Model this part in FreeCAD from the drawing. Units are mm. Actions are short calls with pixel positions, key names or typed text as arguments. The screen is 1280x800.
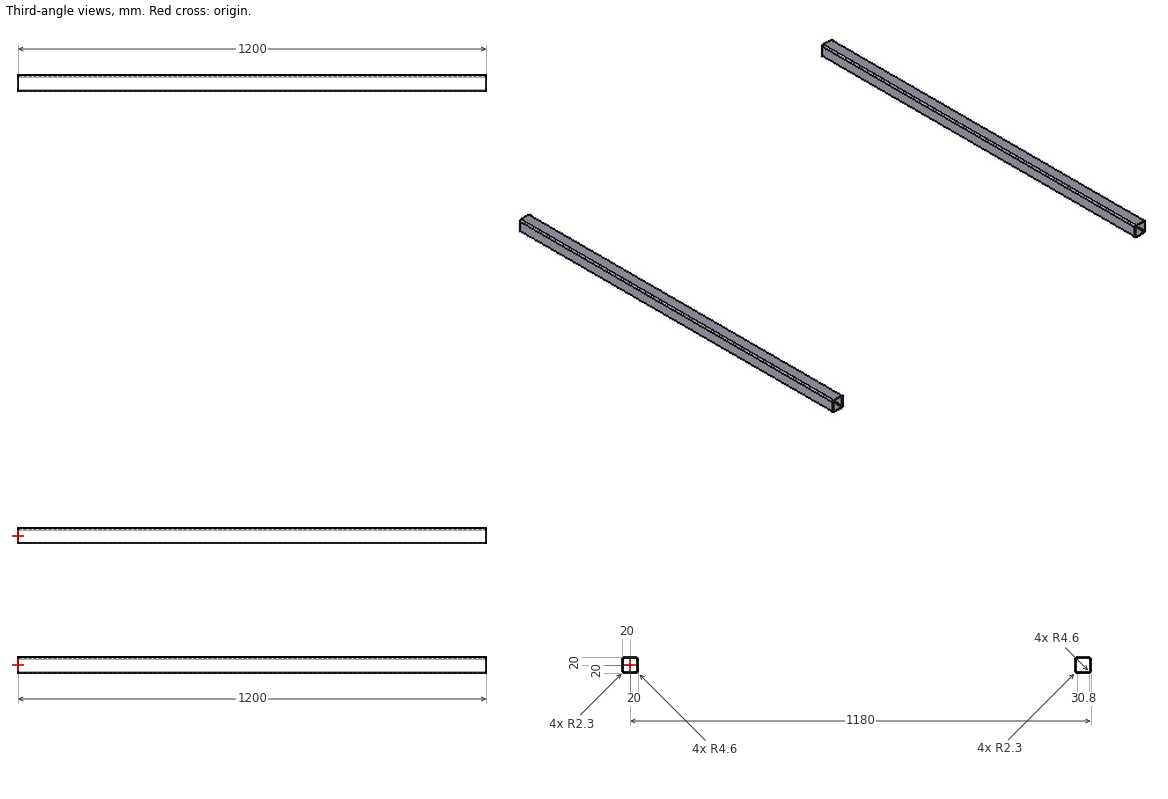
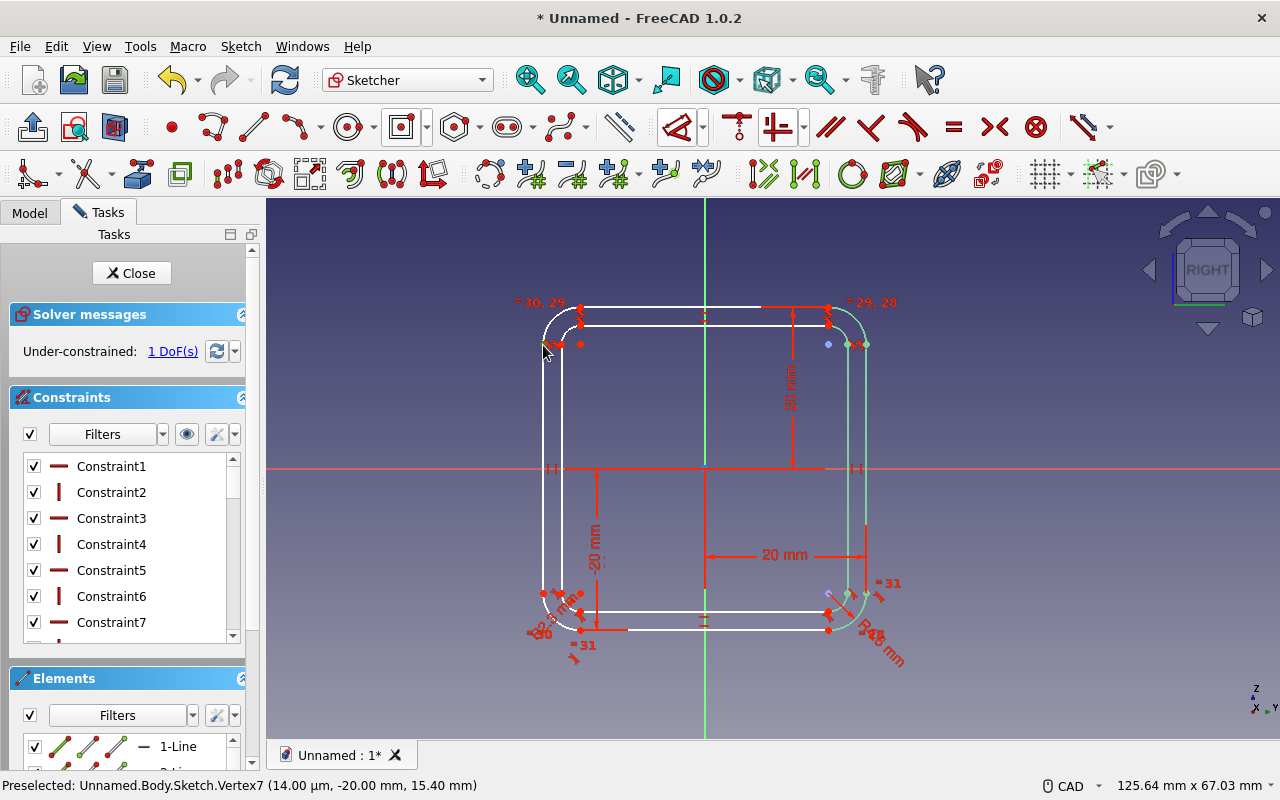
key(l)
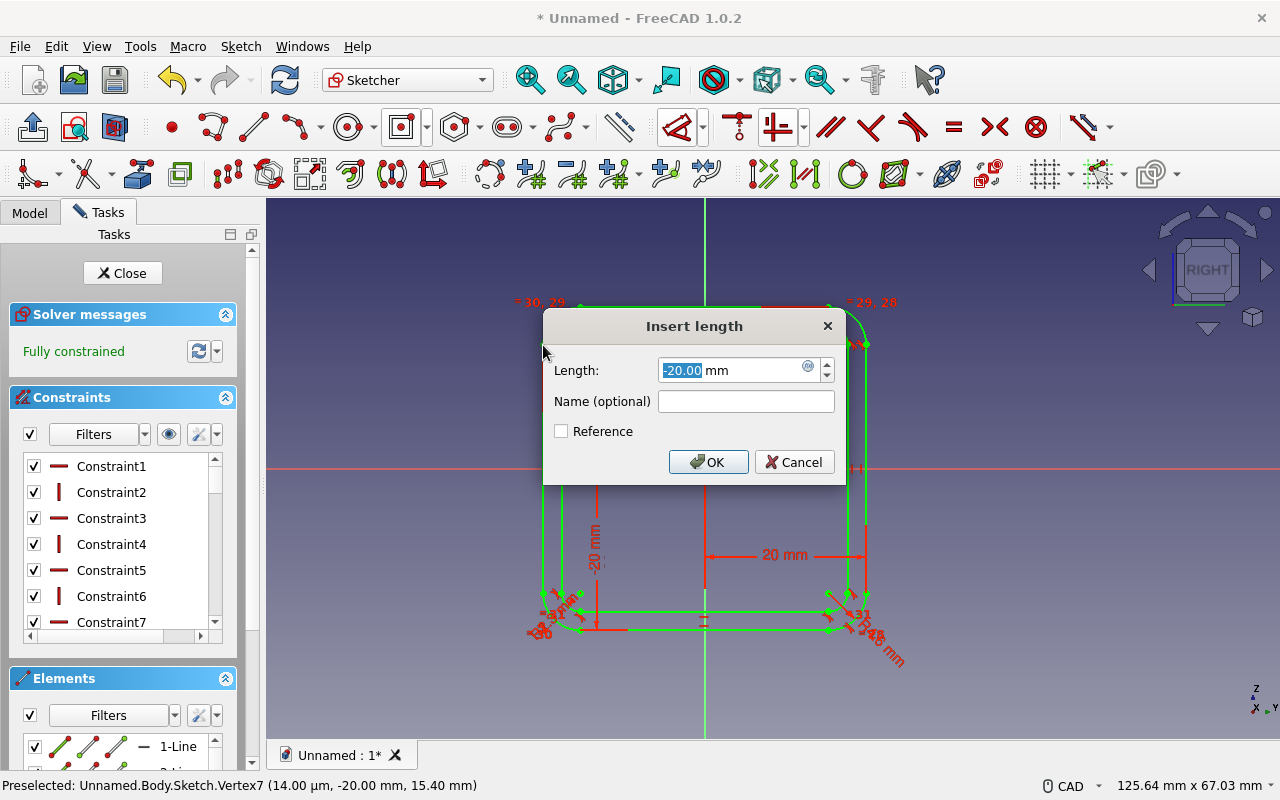
text(-20)
key(Return)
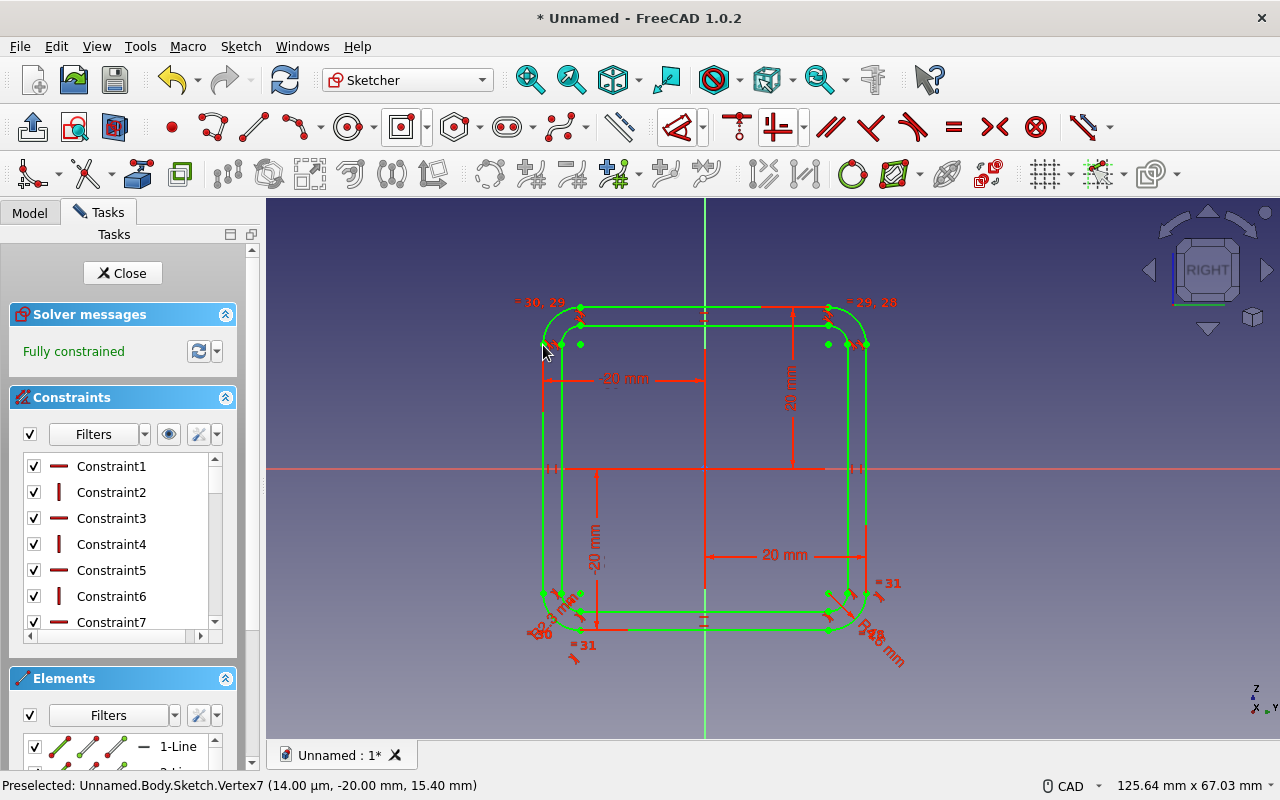
click(123, 273)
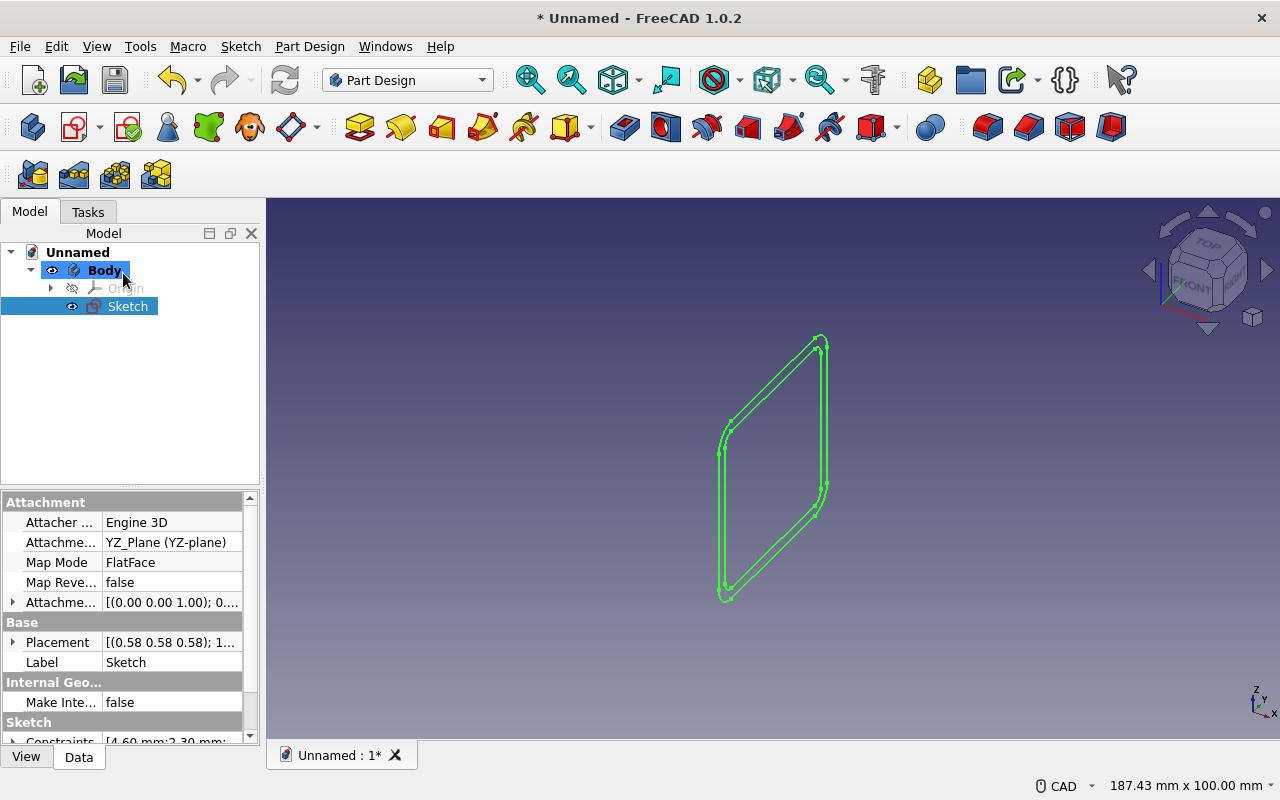
click(360, 128)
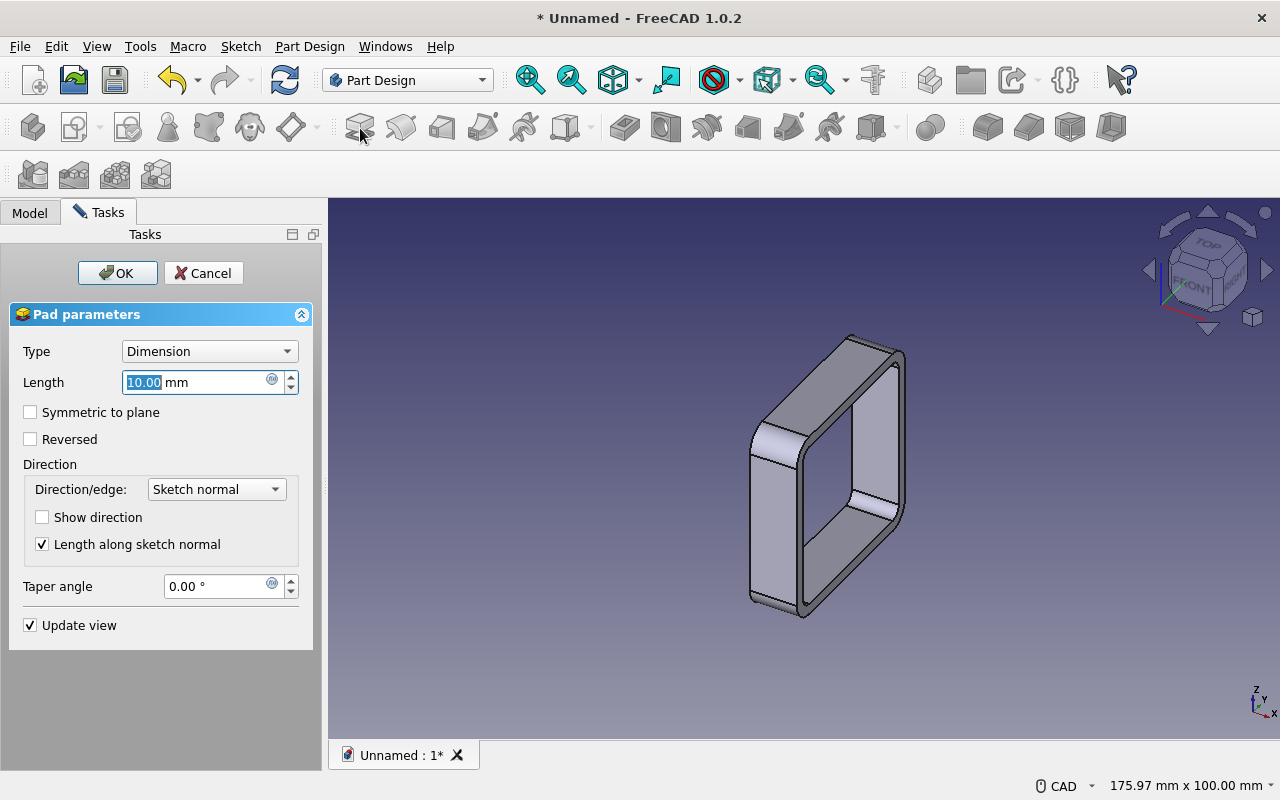
text(1200)
key(Tab)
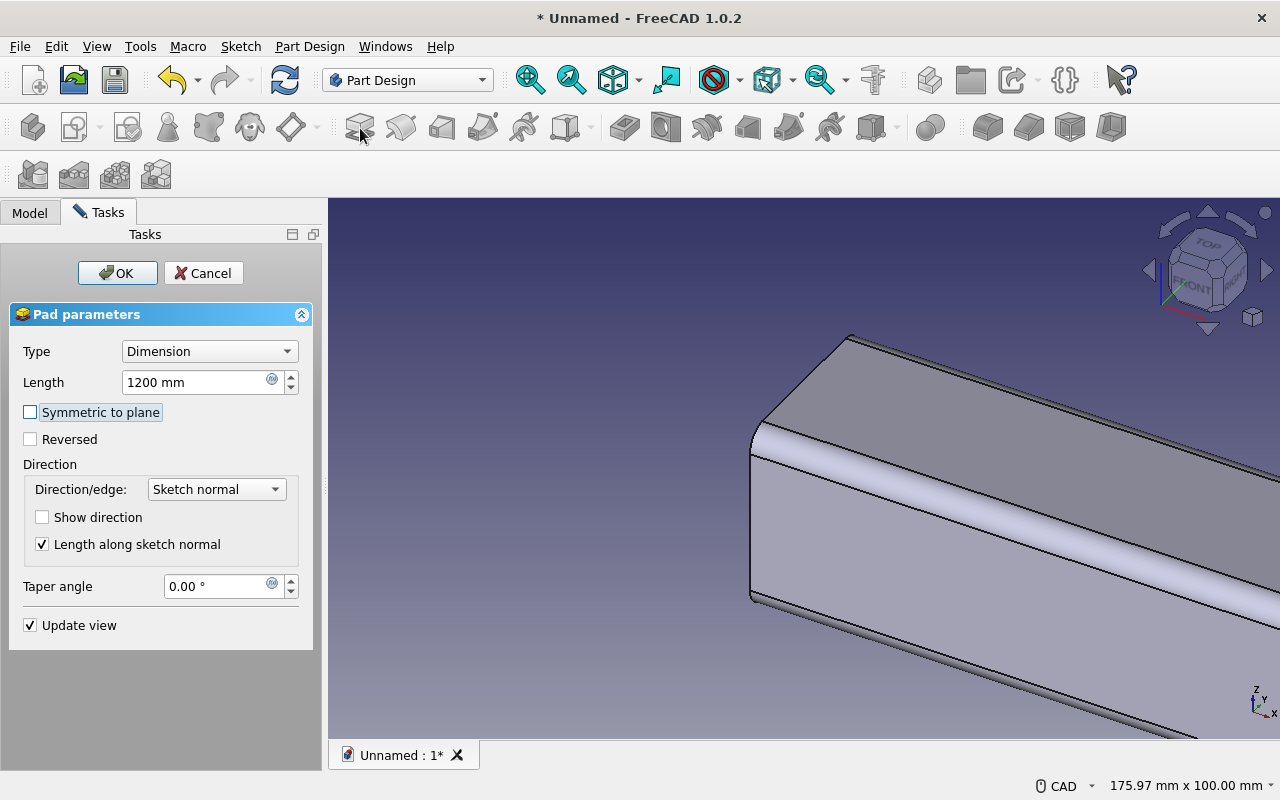
click(118, 273)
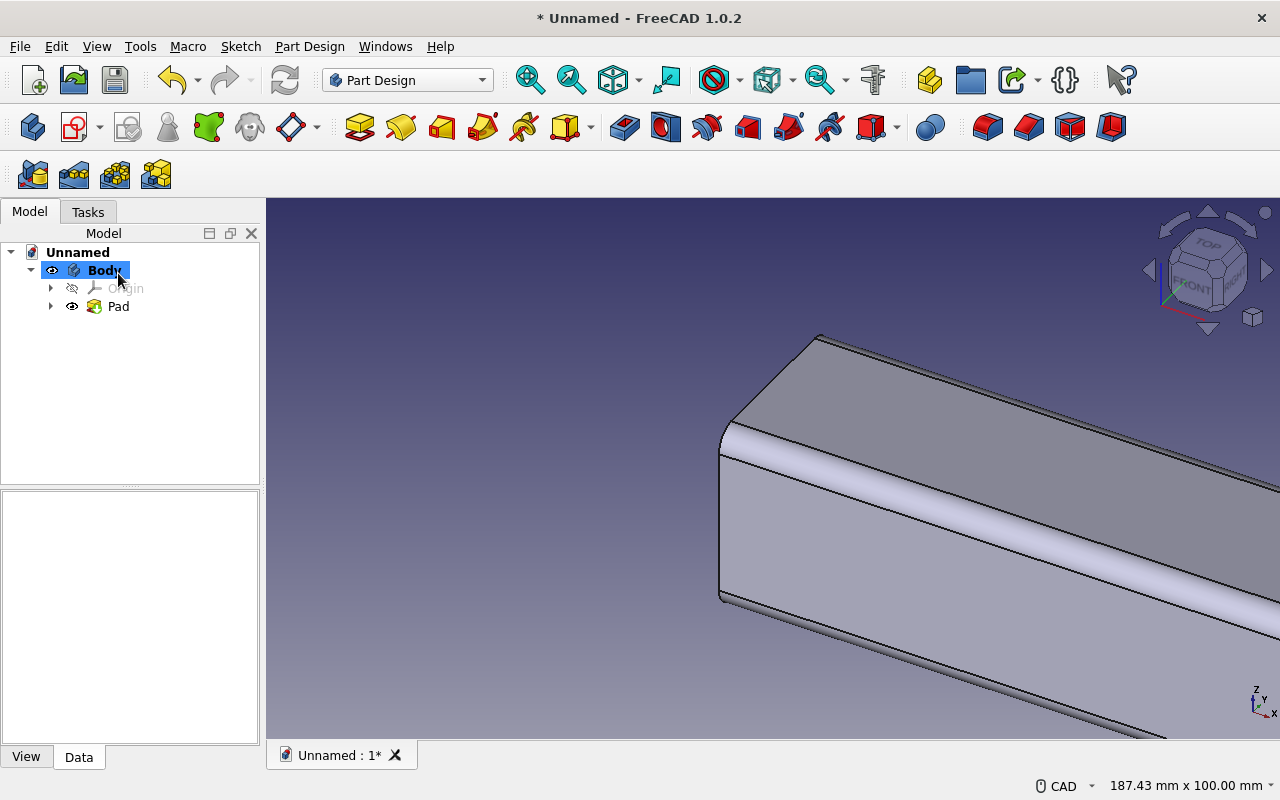
key(v)
key(f)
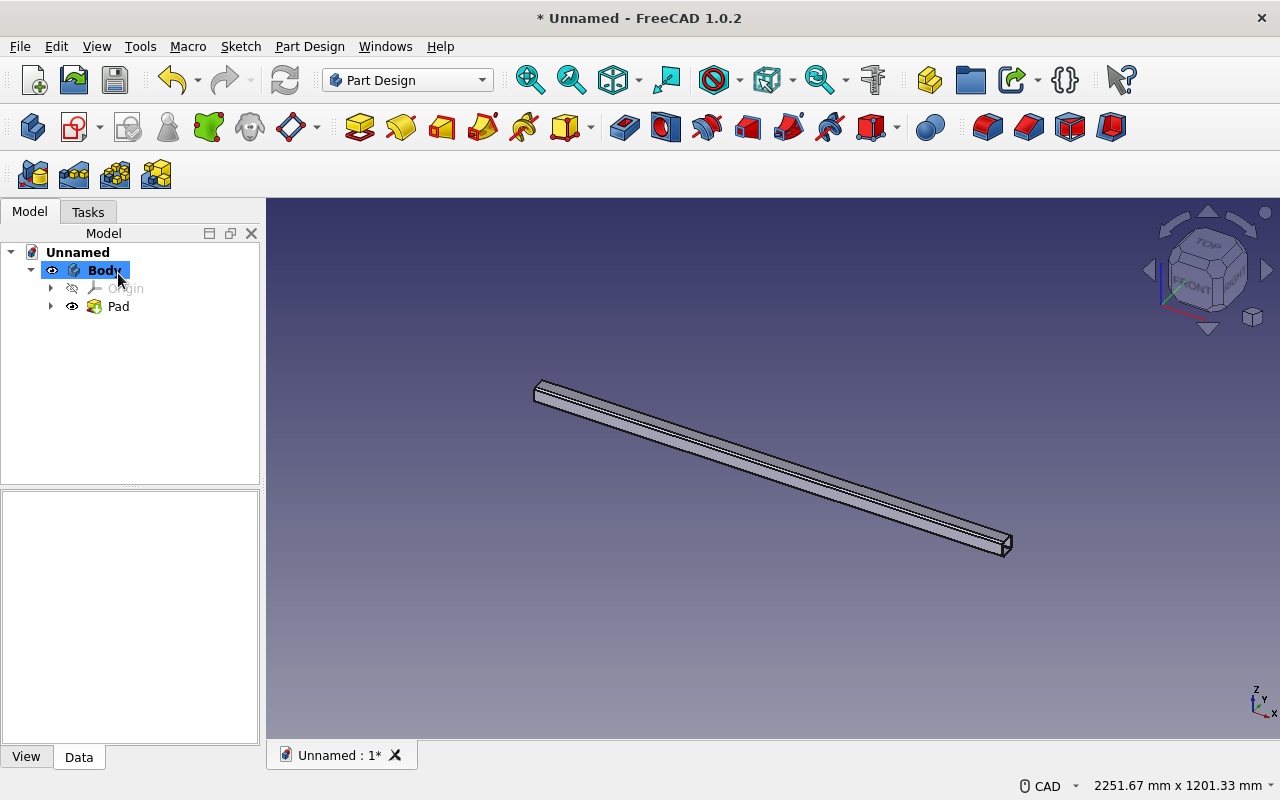
click(33, 128)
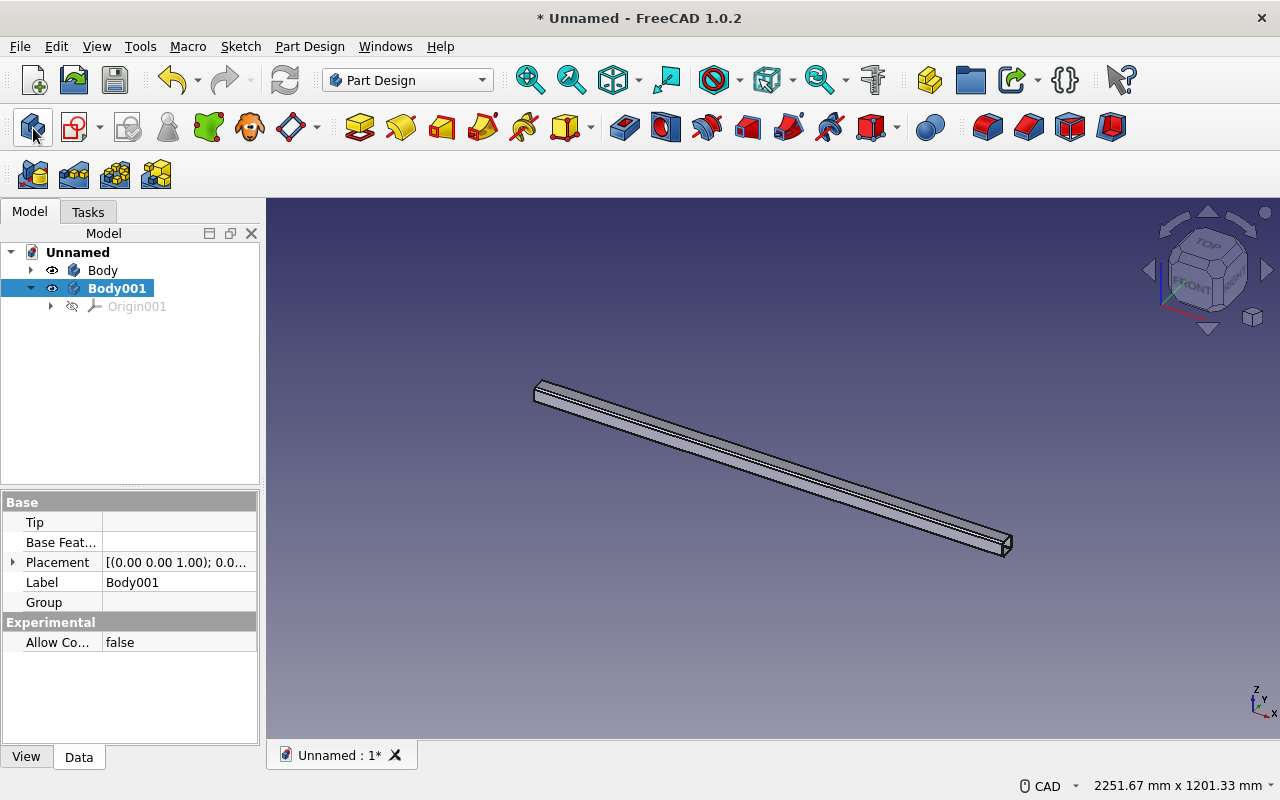
click(306, 699)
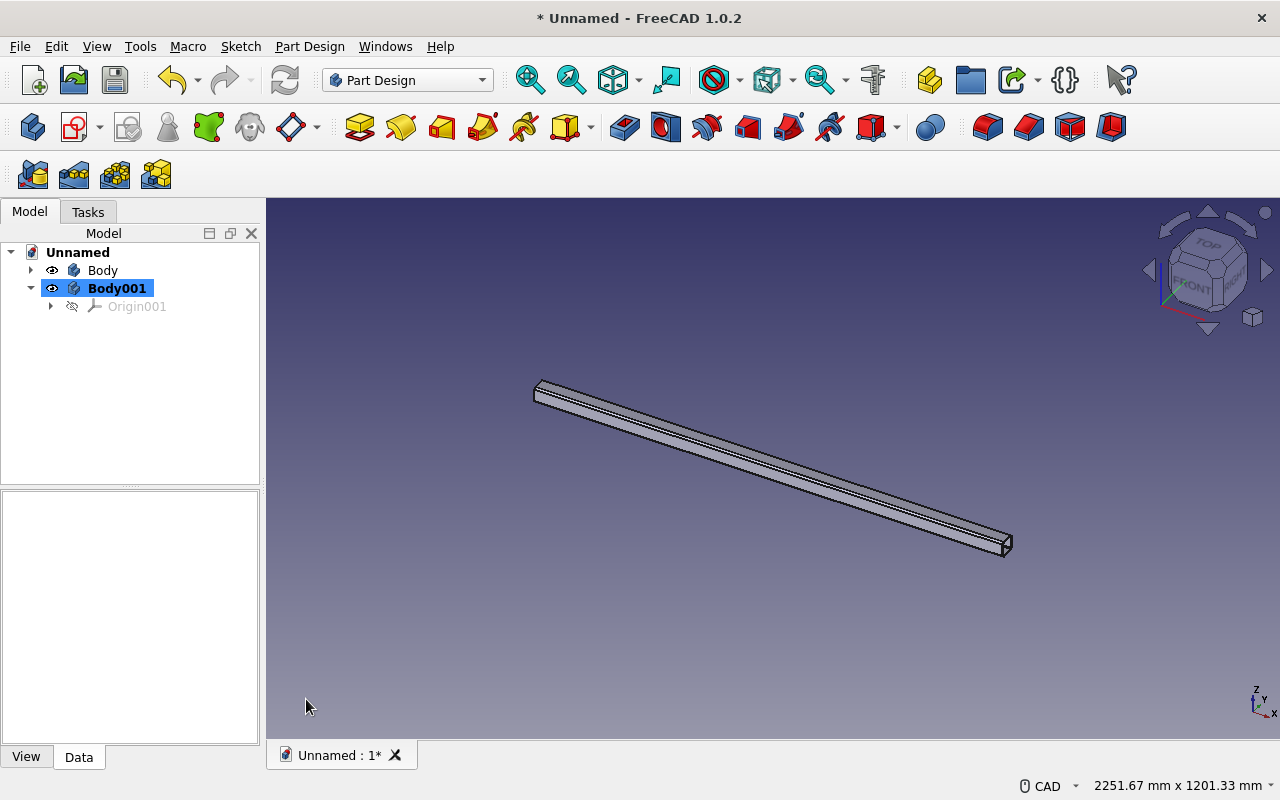
click(74, 128)